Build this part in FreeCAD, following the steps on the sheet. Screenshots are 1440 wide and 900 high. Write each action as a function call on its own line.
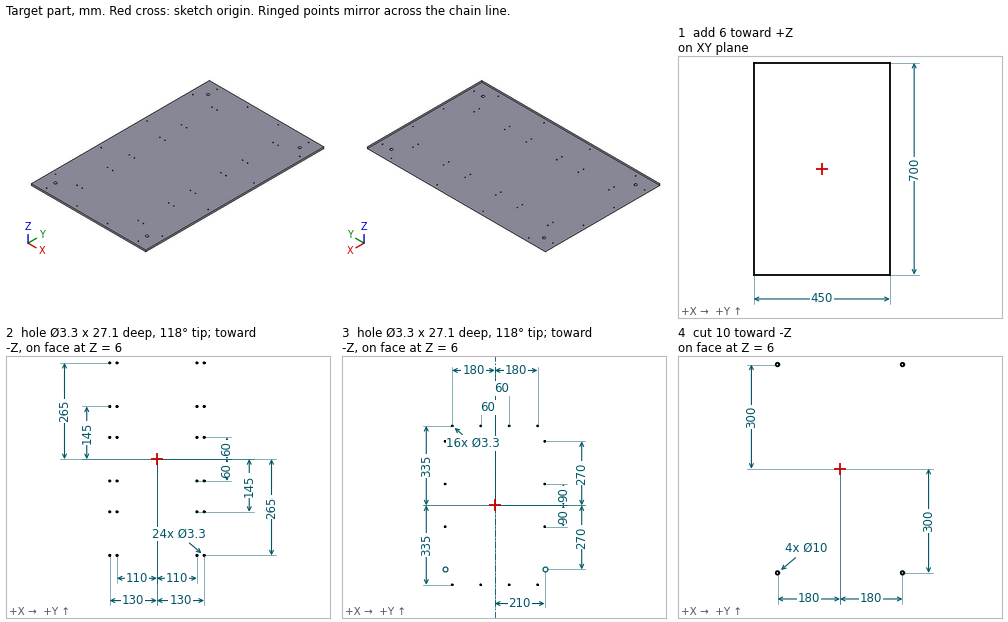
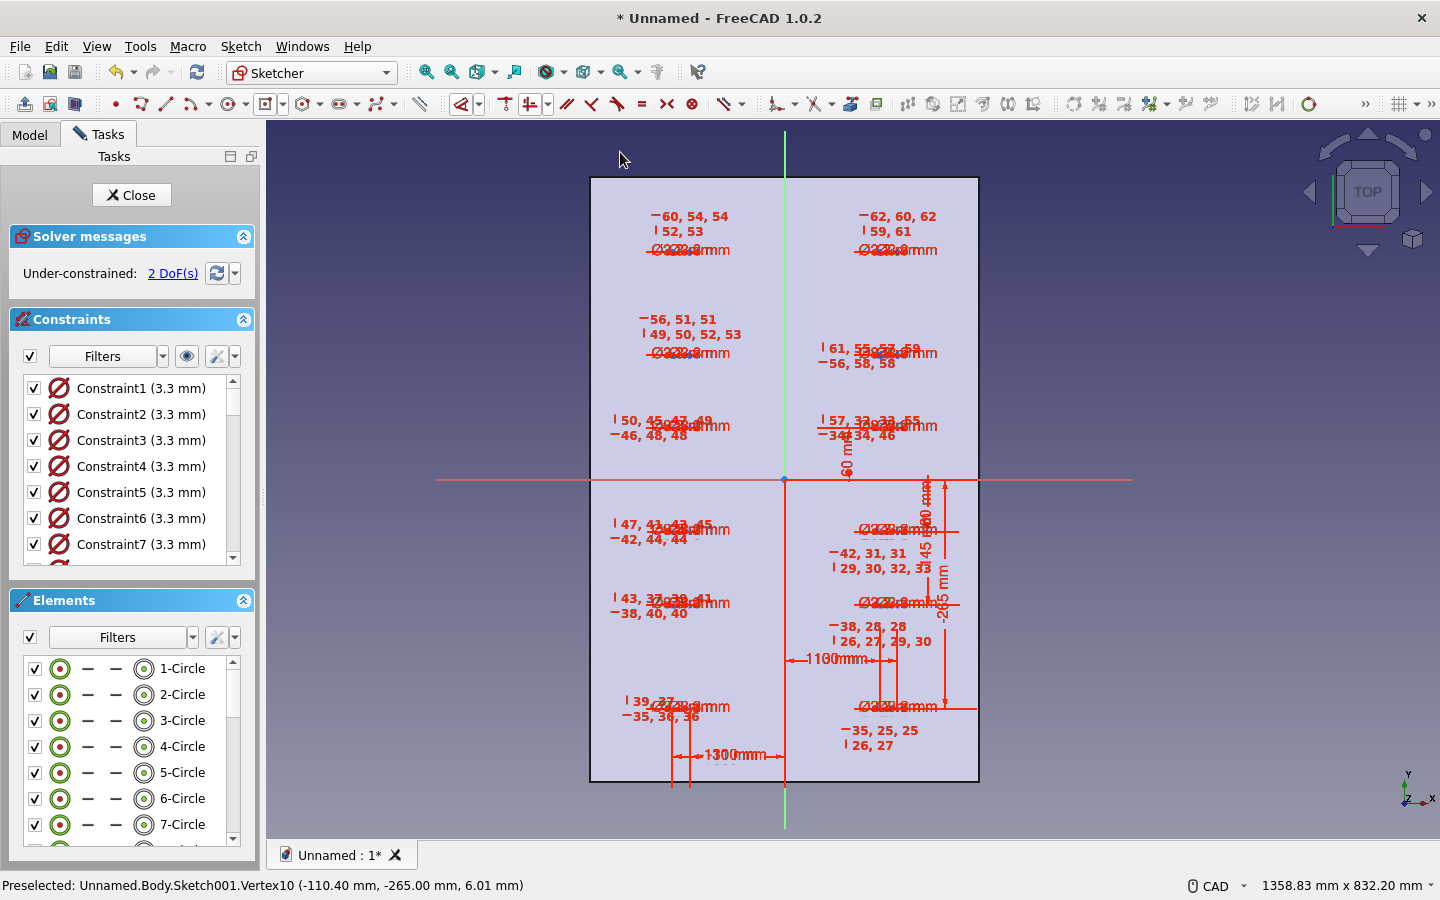
click(672, 355)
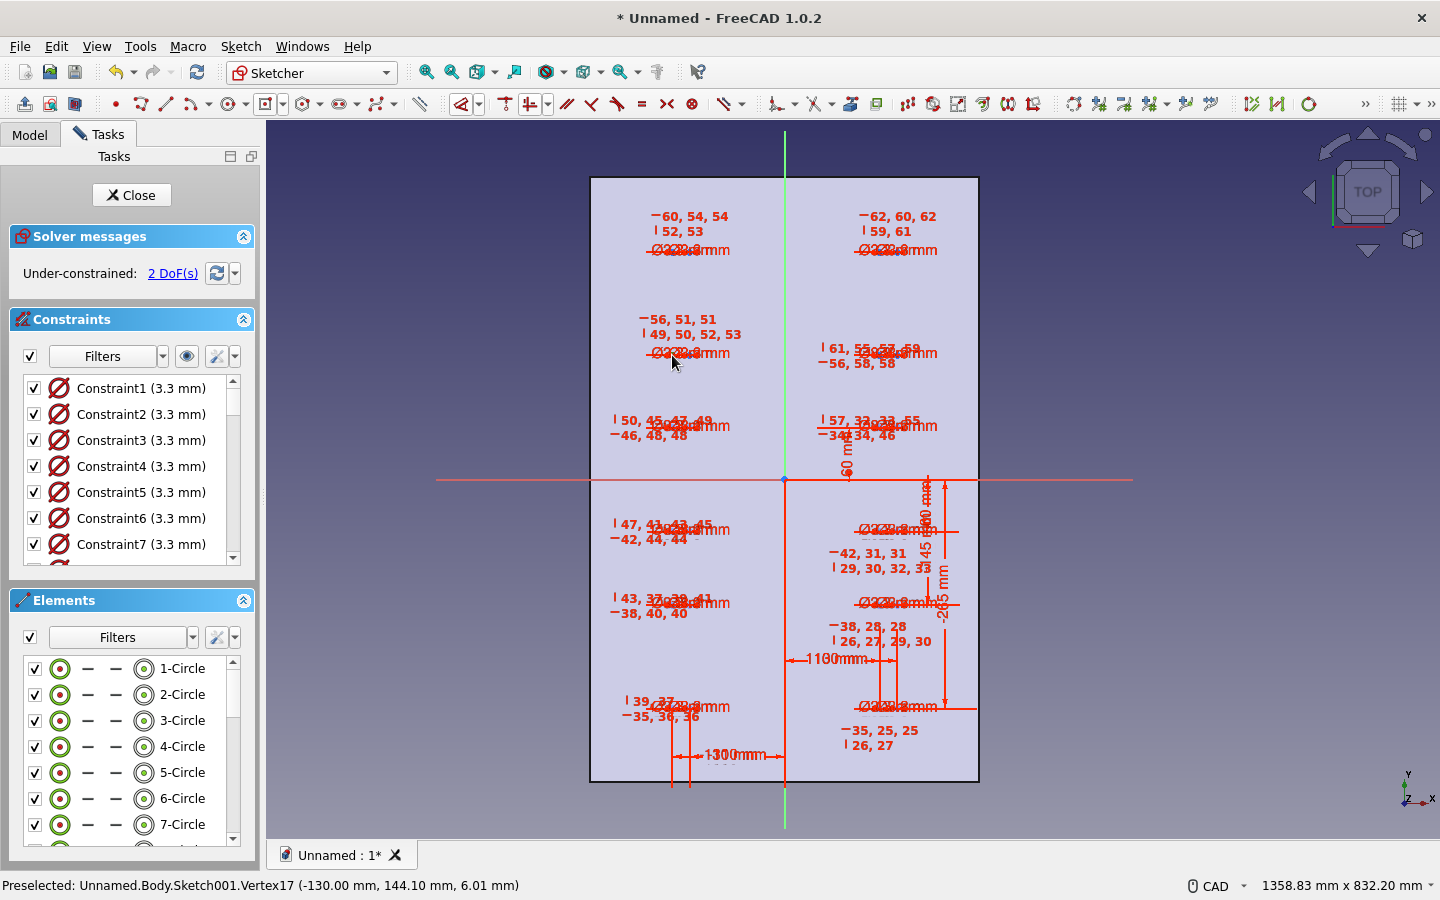
click(478, 104)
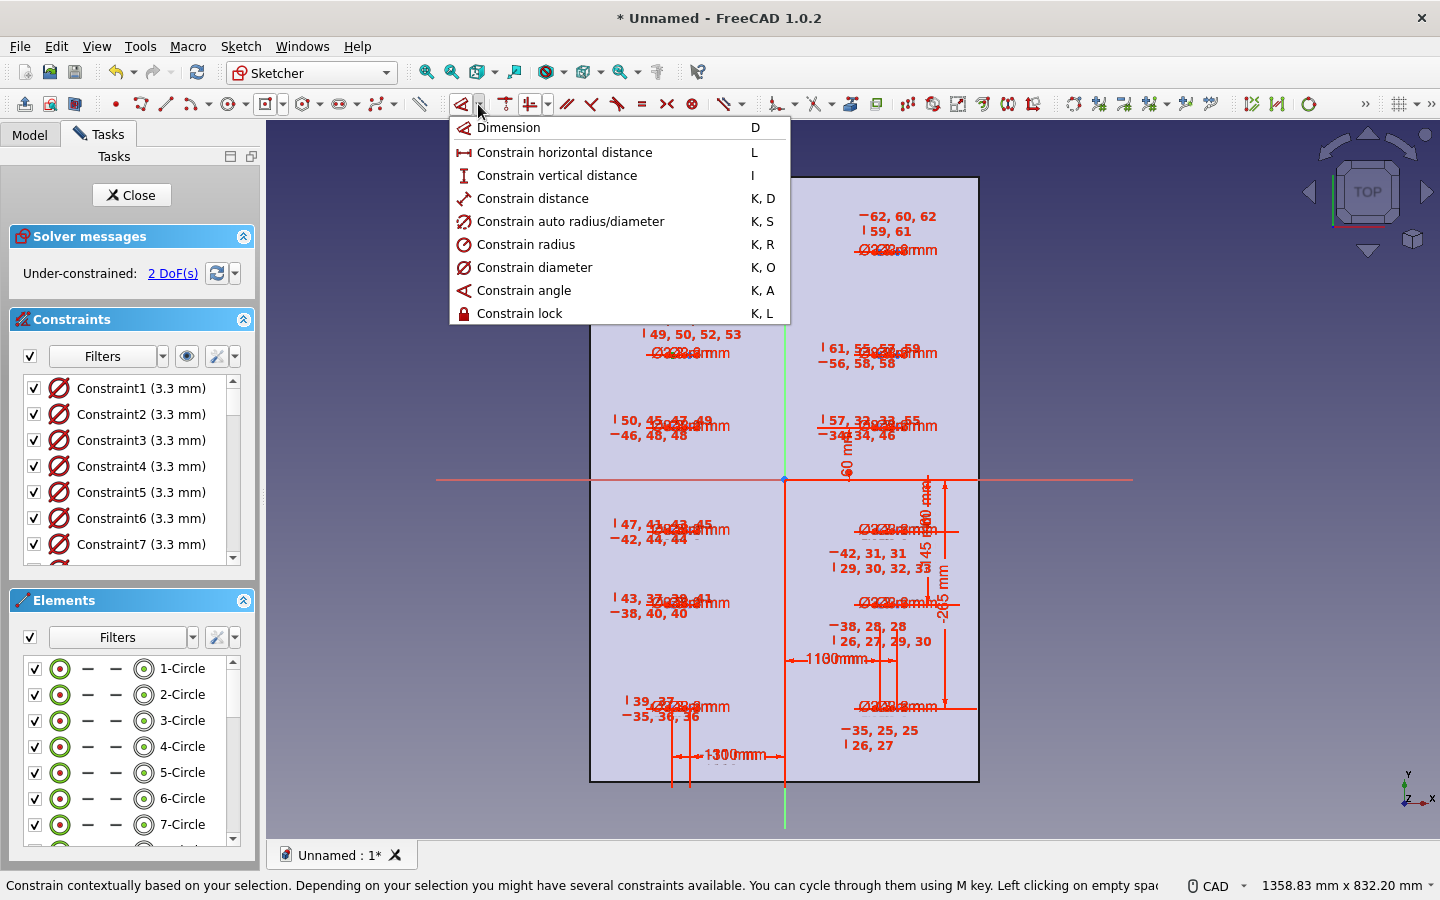
click(620, 176)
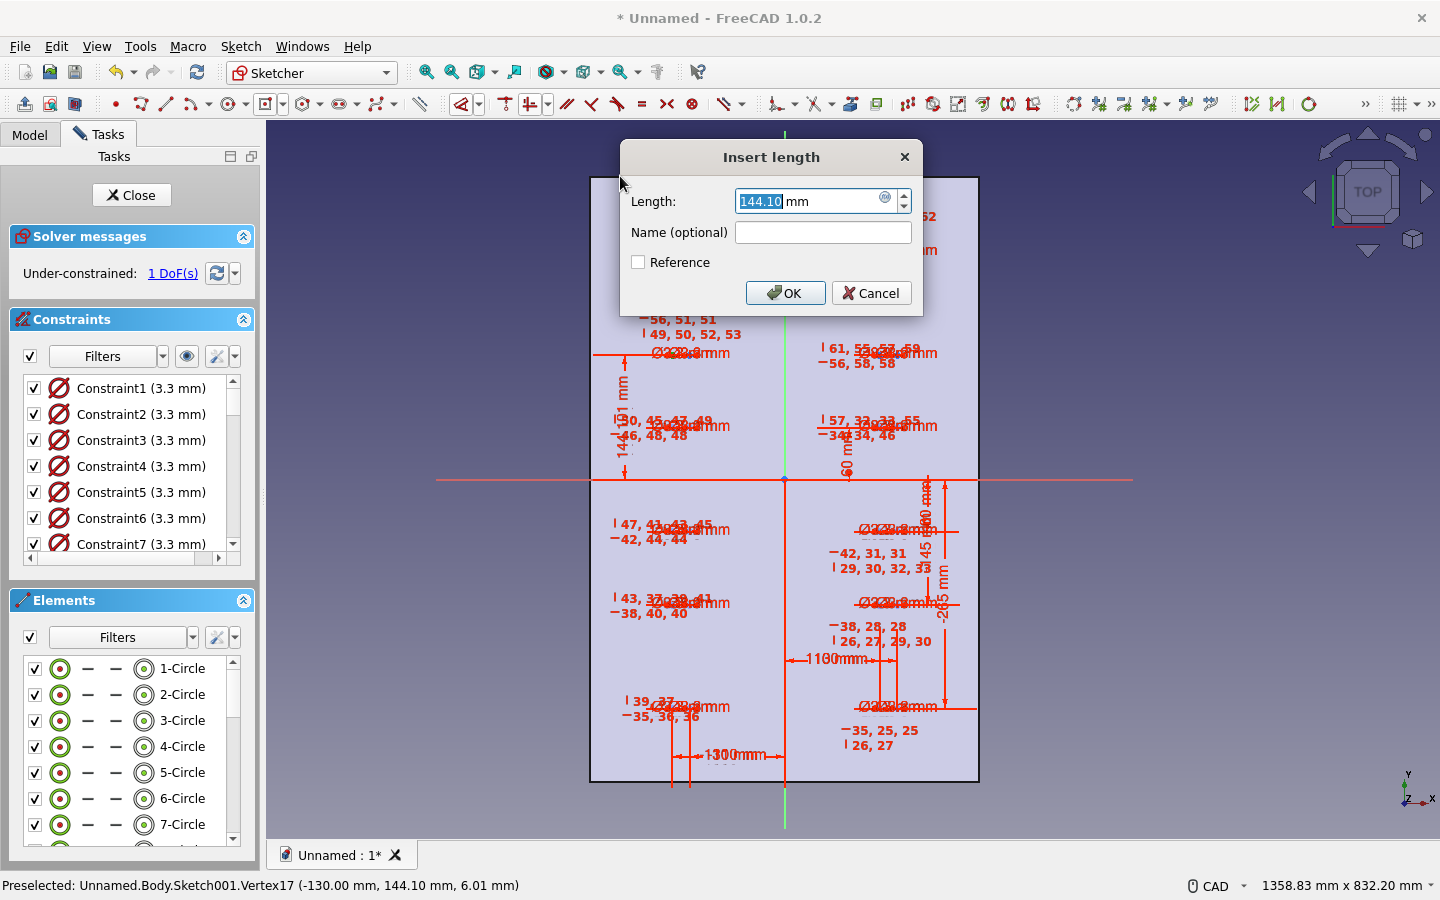
text(145)
key(Return)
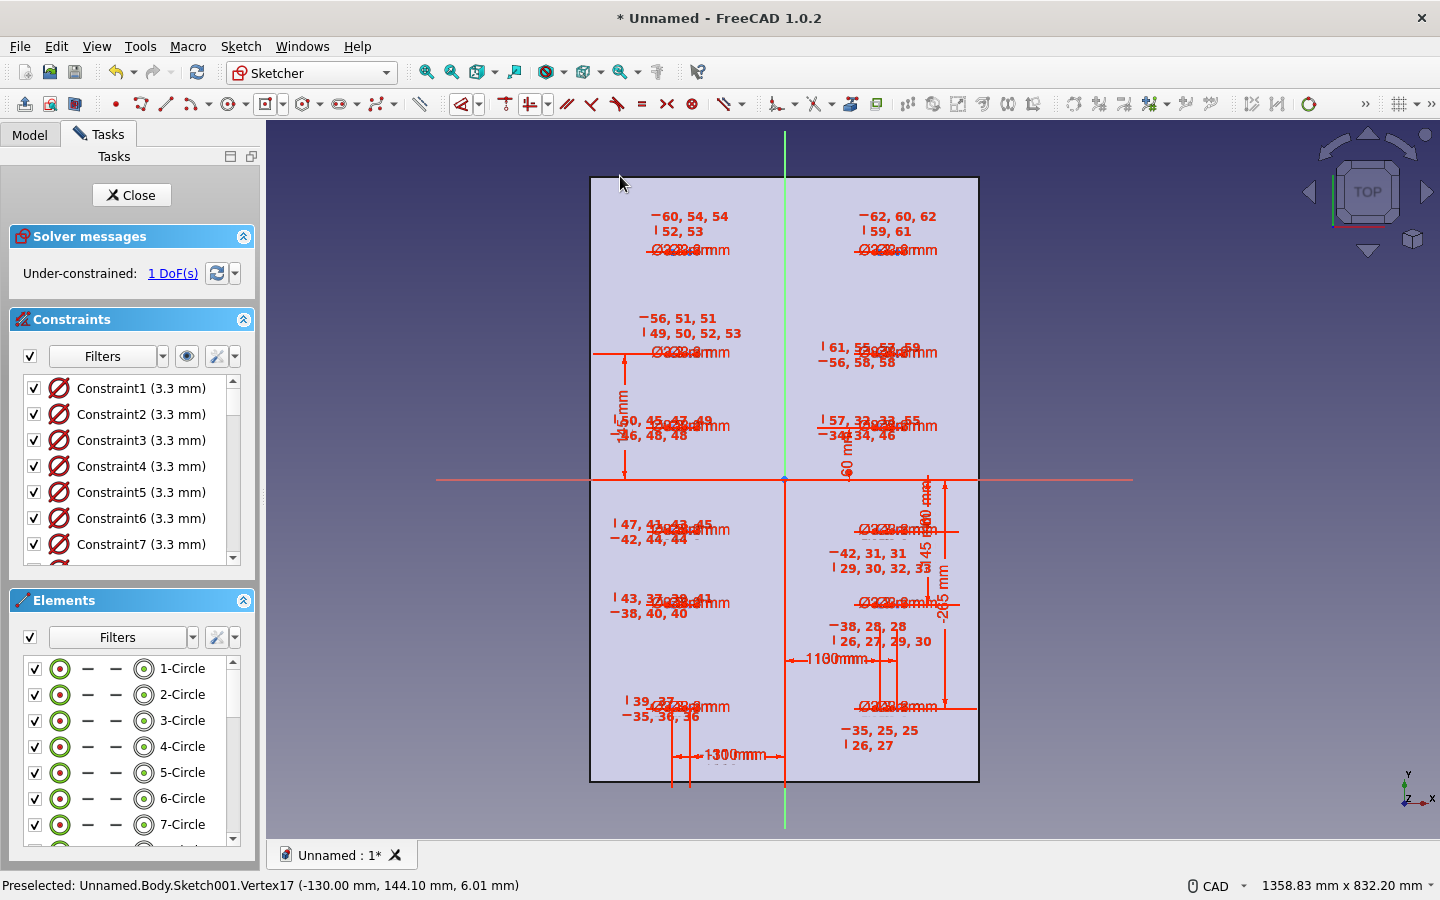
click(672, 252)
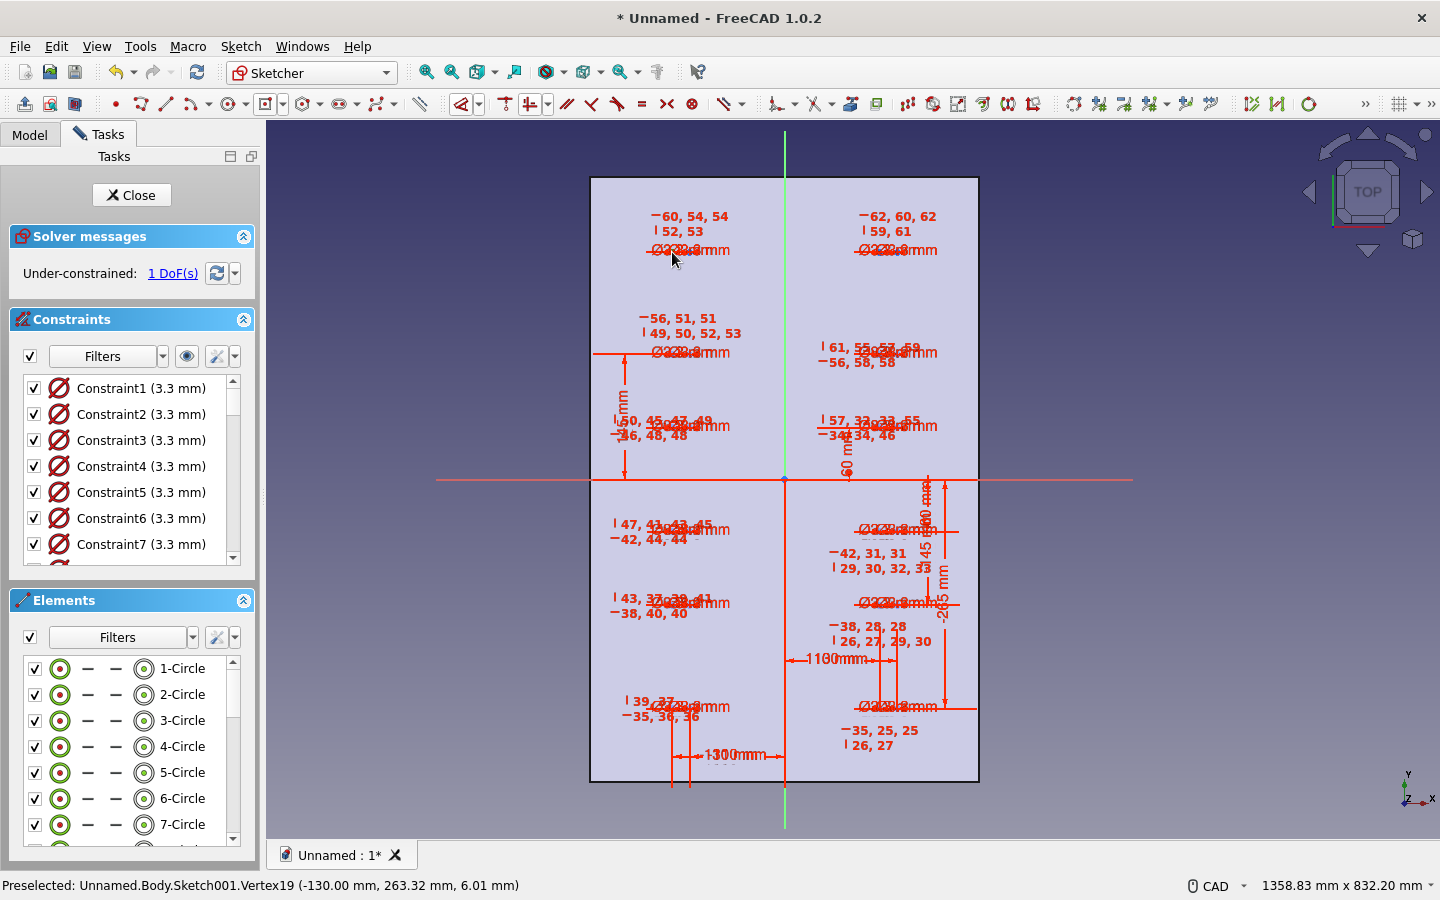
key(i)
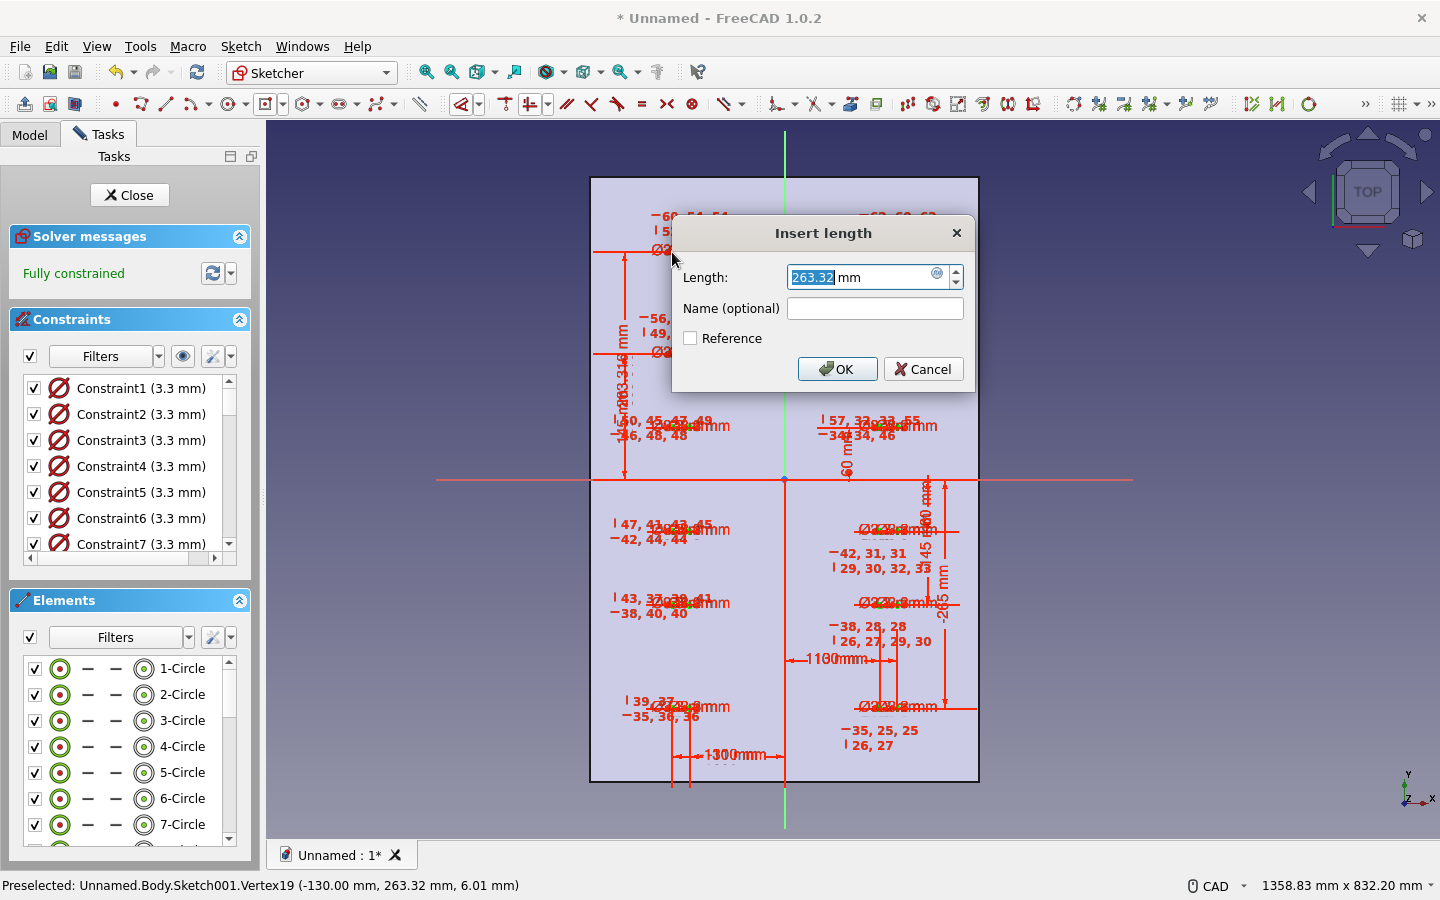
text(265)
key(Return)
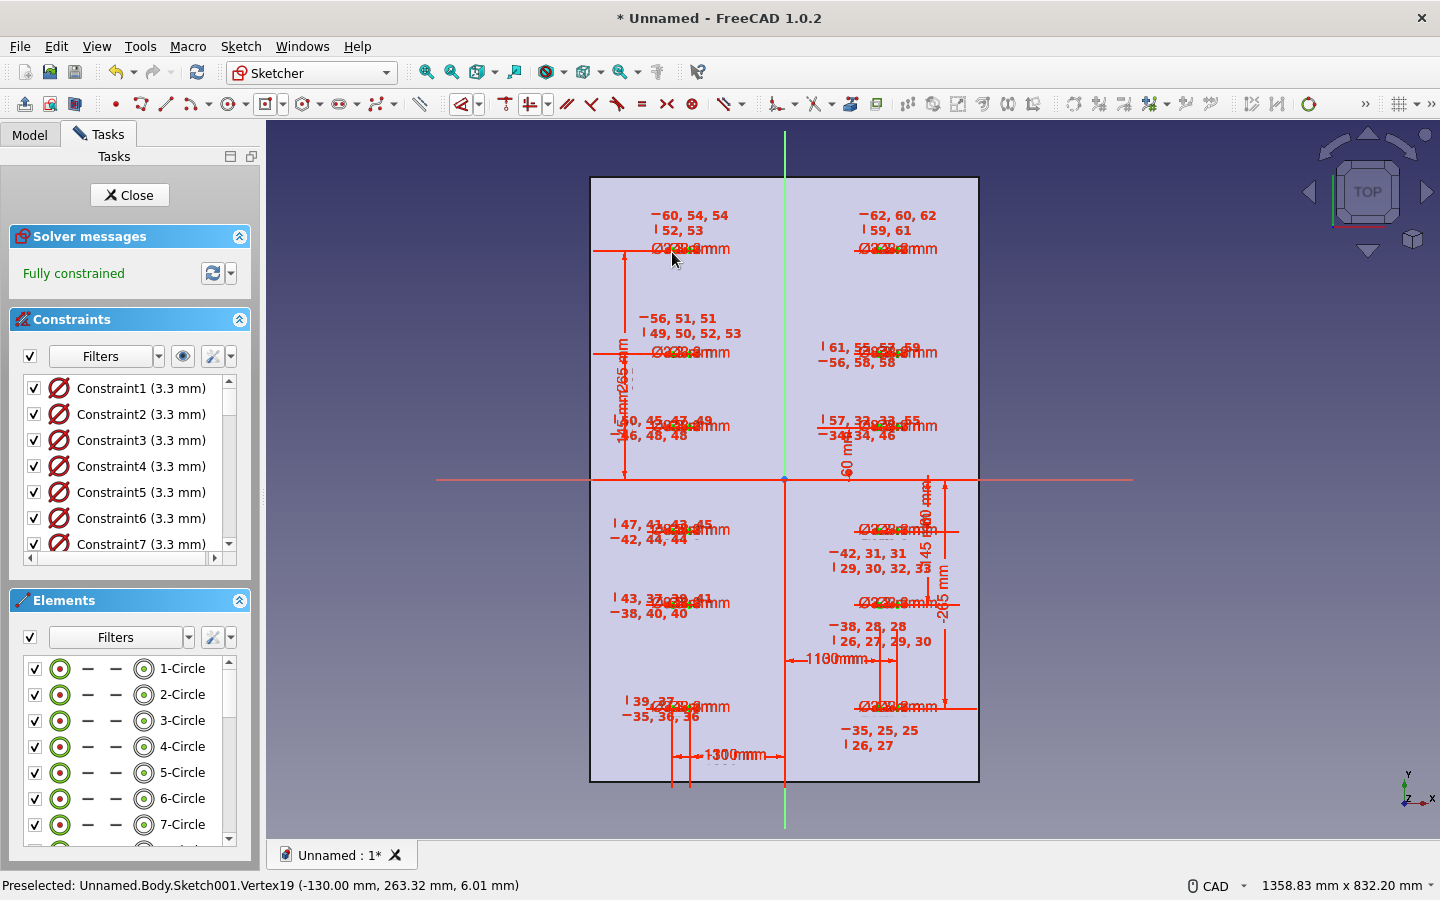
click(130, 195)